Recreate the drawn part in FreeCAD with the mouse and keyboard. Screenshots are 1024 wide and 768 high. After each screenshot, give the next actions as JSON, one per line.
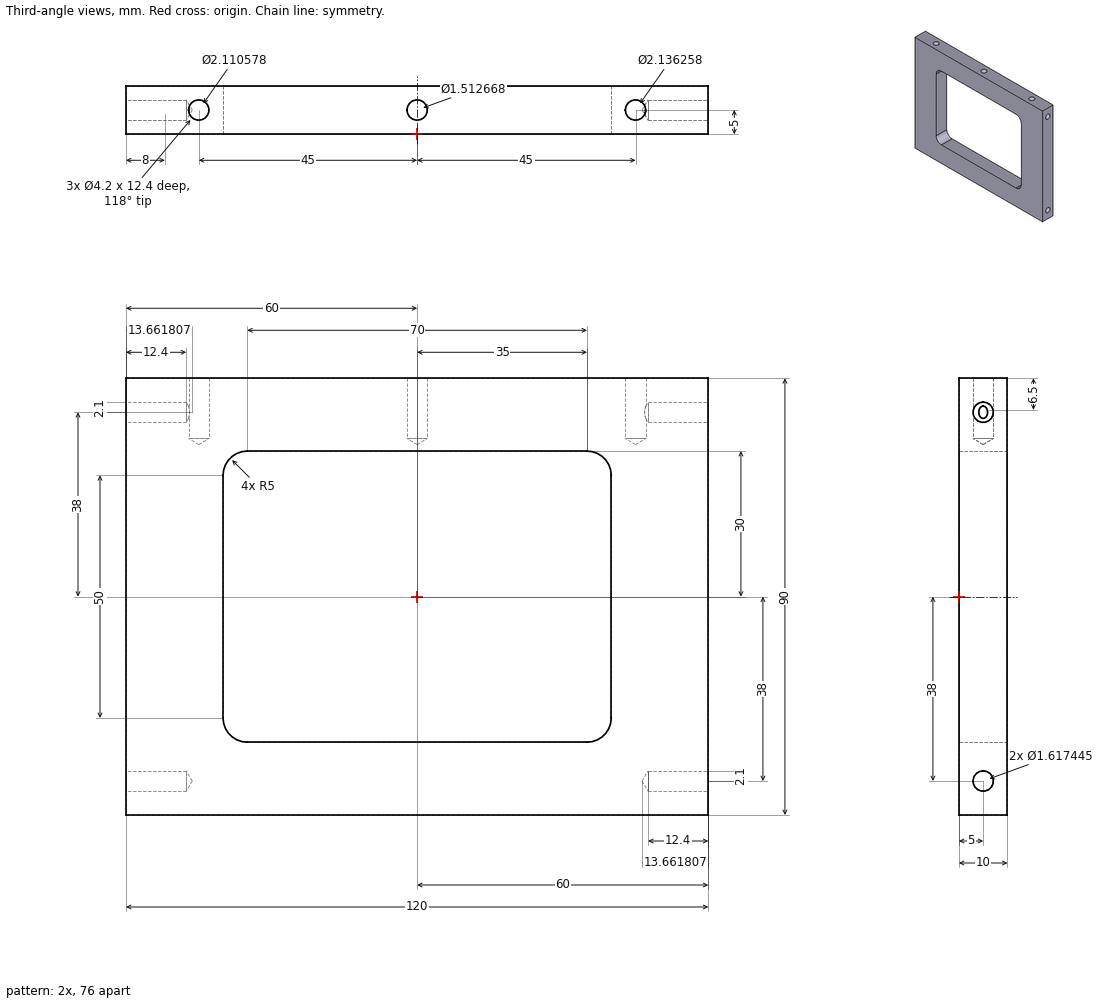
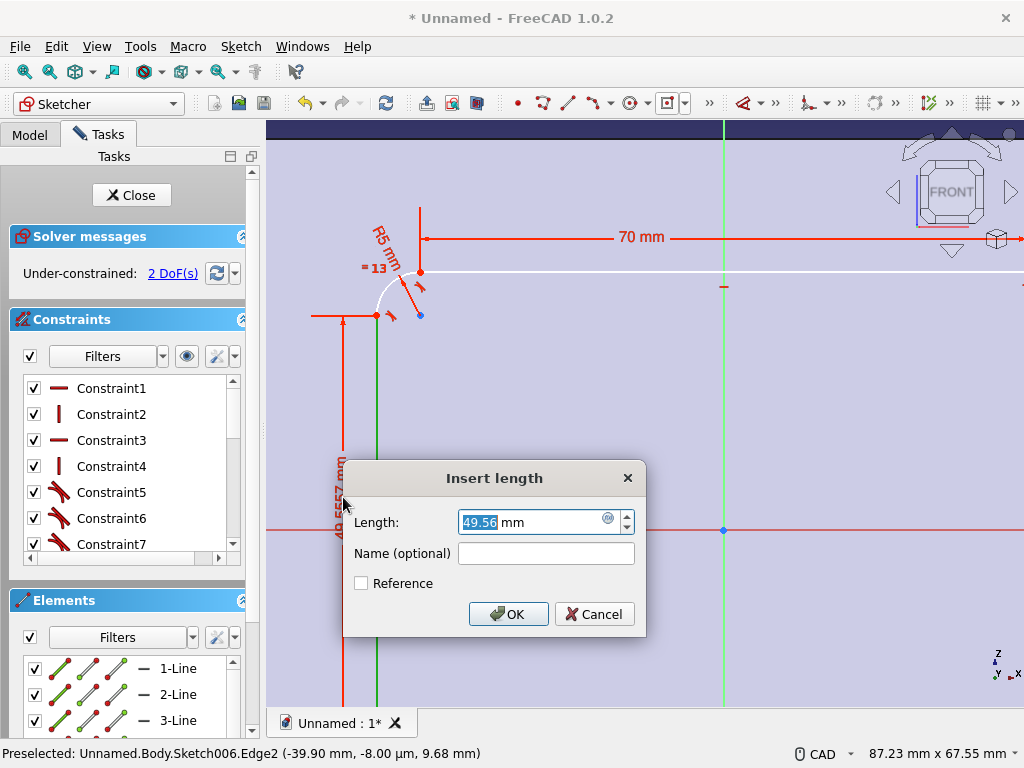
{"action": "type", "text": "50"}
{"action": "key", "text": "Return"}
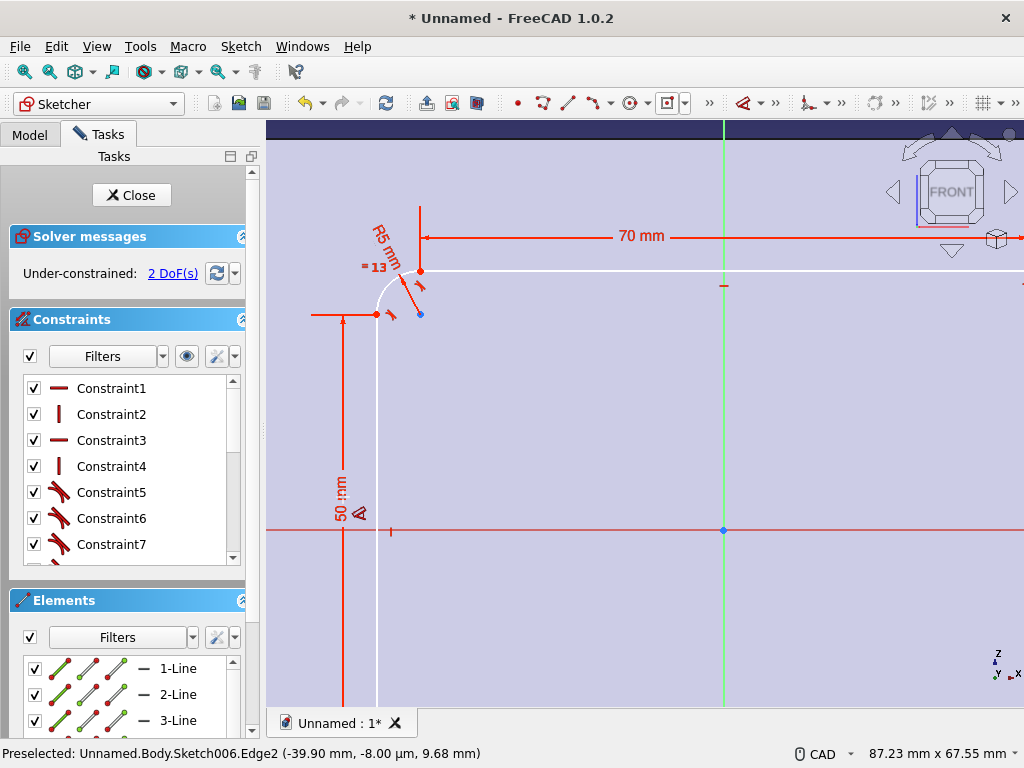
{"action": "scroll", "coordinate": [398, 272], "scroll_direction": "down", "scroll_amount": 3}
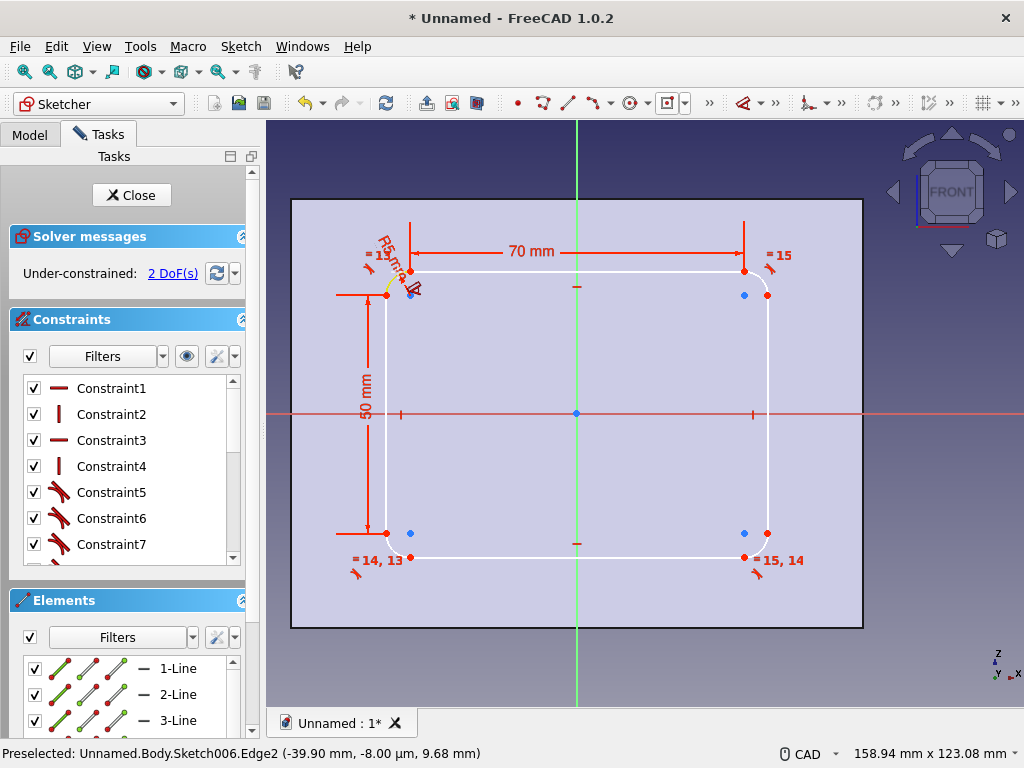
{"action": "left_click", "coordinate": [744, 272]}
{"action": "left_click", "coordinate": [660, 238]}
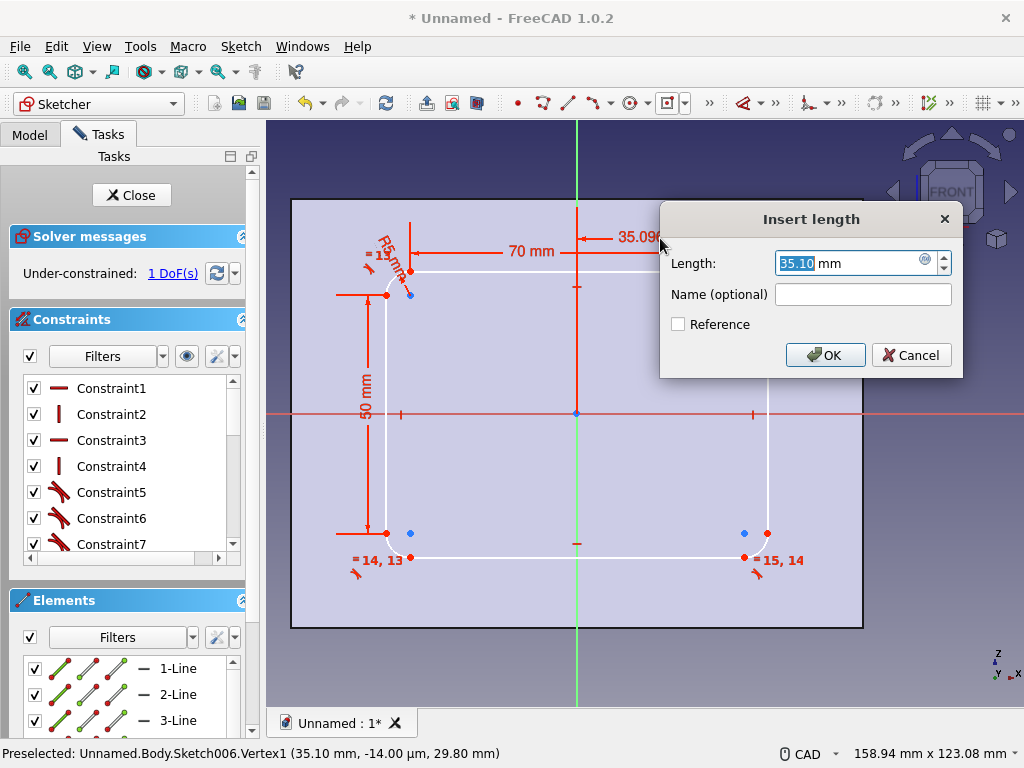
{"action": "type", "text": "35"}
{"action": "key", "text": "Return"}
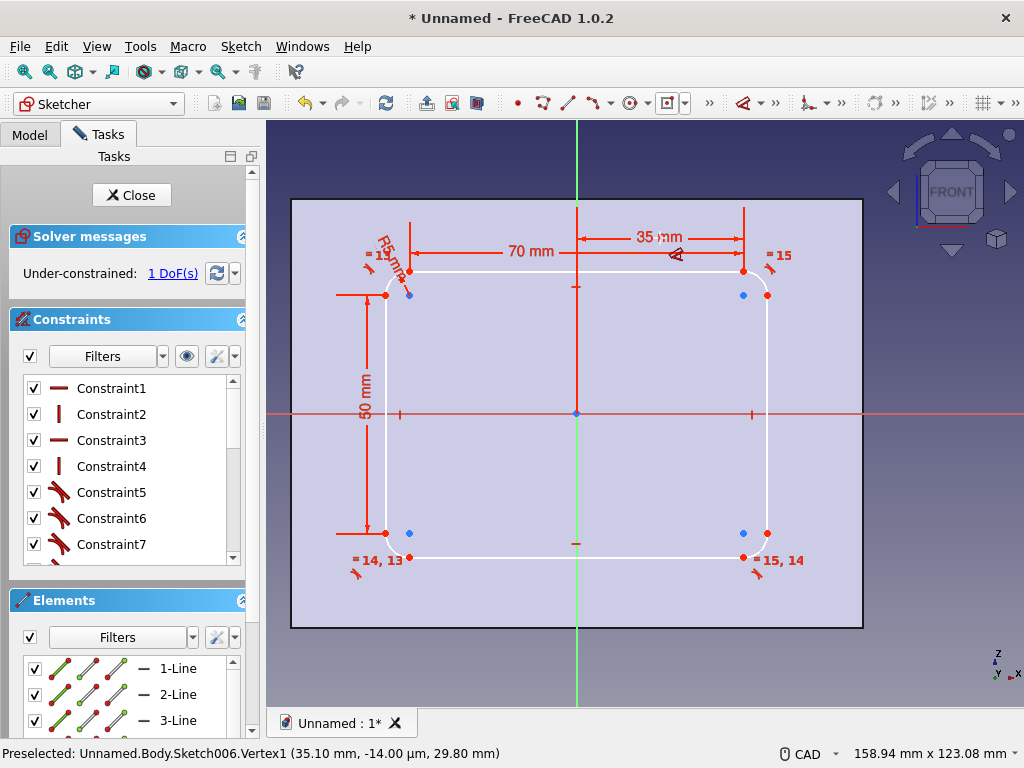
{"action": "left_click", "coordinate": [744, 272]}
{"action": "left_click", "coordinate": [543, 343]}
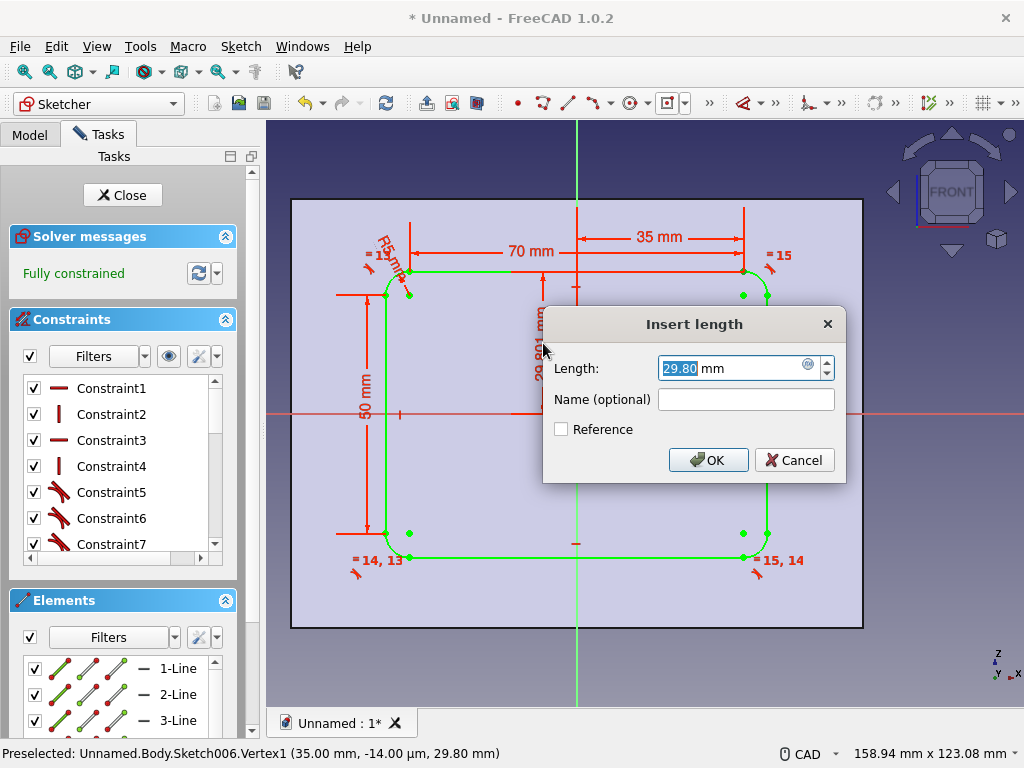
{"action": "type", "text": "30"}
{"action": "key", "text": "Return"}
{"action": "key", "text": "Escape"}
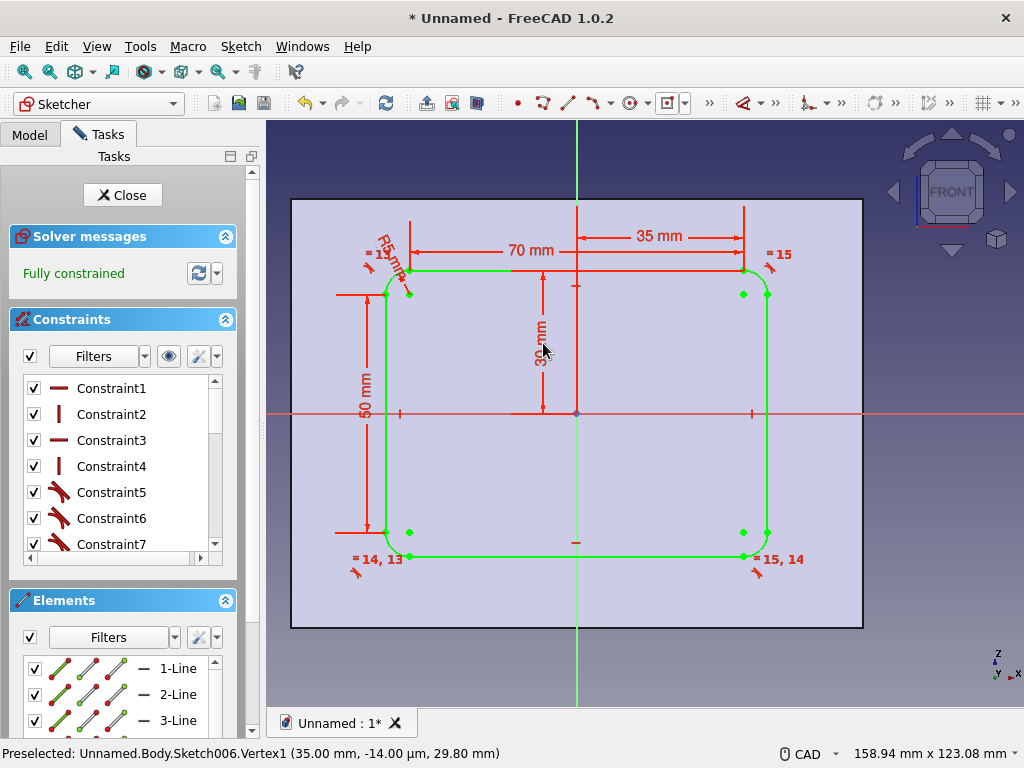
{"action": "left_click", "coordinate": [123, 195]}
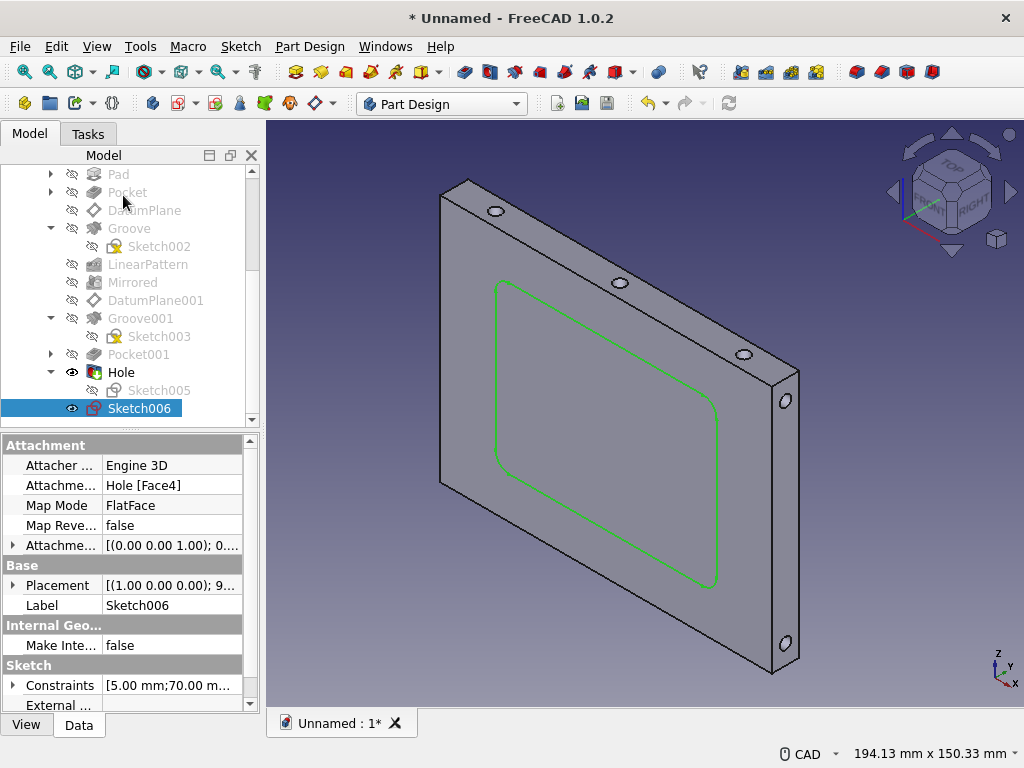
{"action": "left_click", "coordinate": [465, 72]}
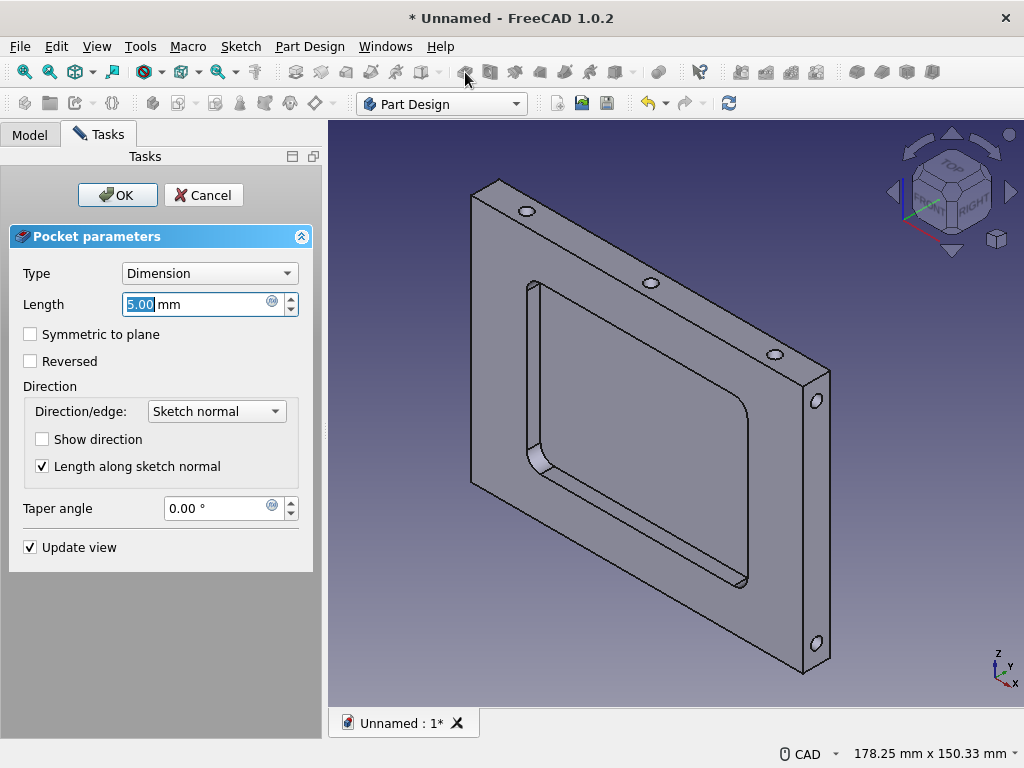
{"action": "left_click", "coordinate": [210, 274]}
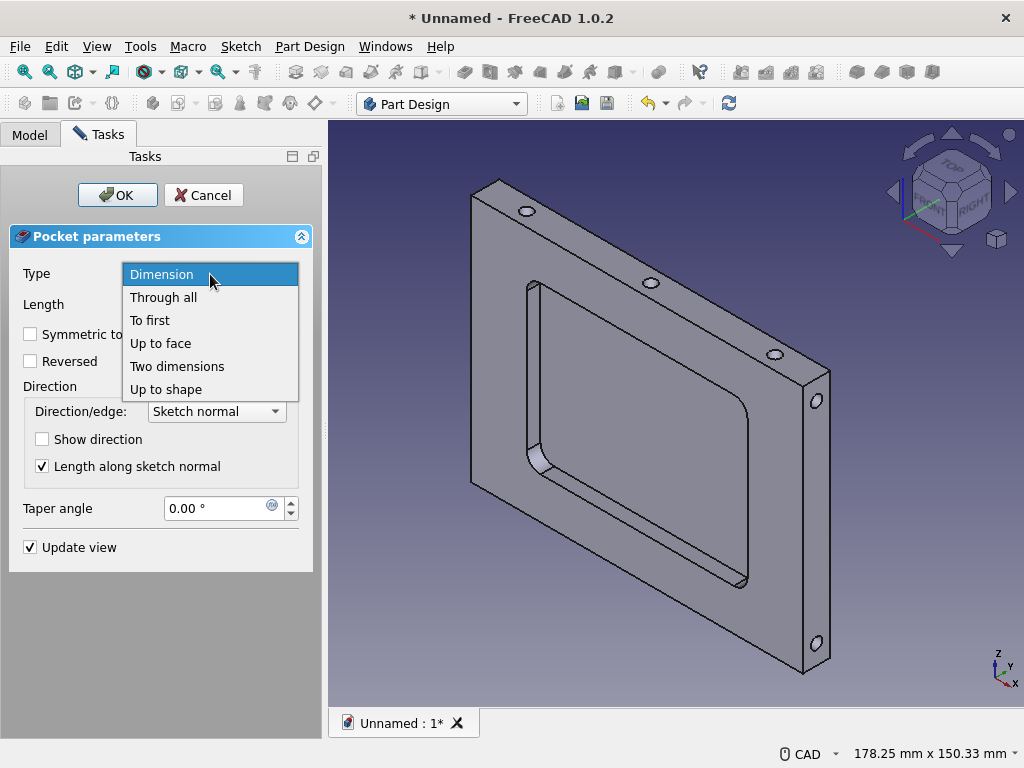
{"action": "left_click", "coordinate": [208, 298]}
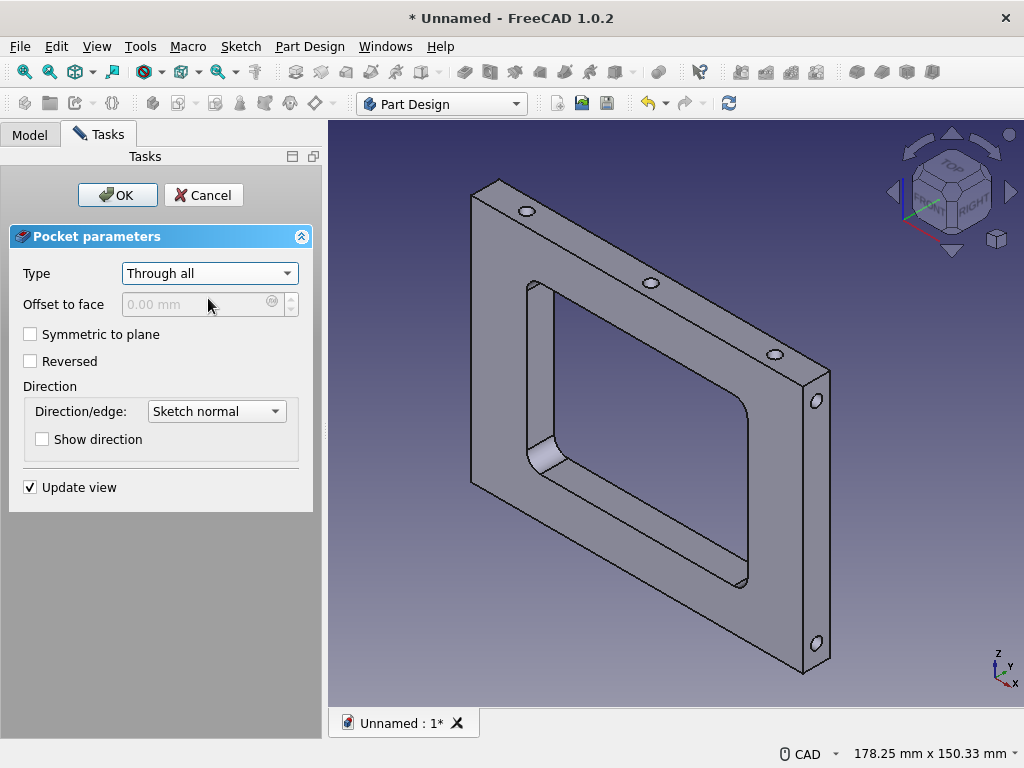
{"action": "left_click", "coordinate": [118, 195]}